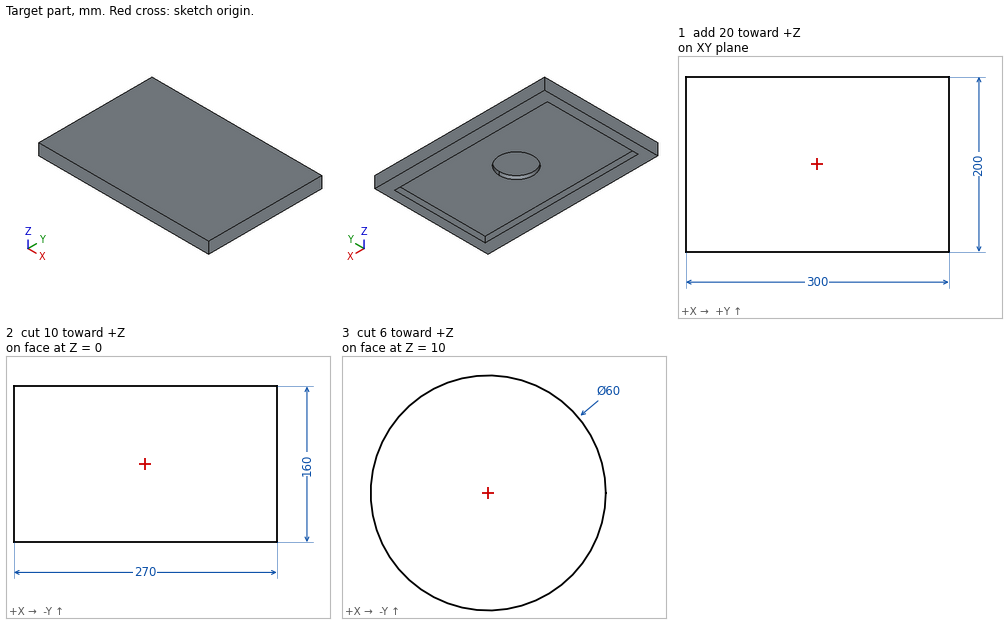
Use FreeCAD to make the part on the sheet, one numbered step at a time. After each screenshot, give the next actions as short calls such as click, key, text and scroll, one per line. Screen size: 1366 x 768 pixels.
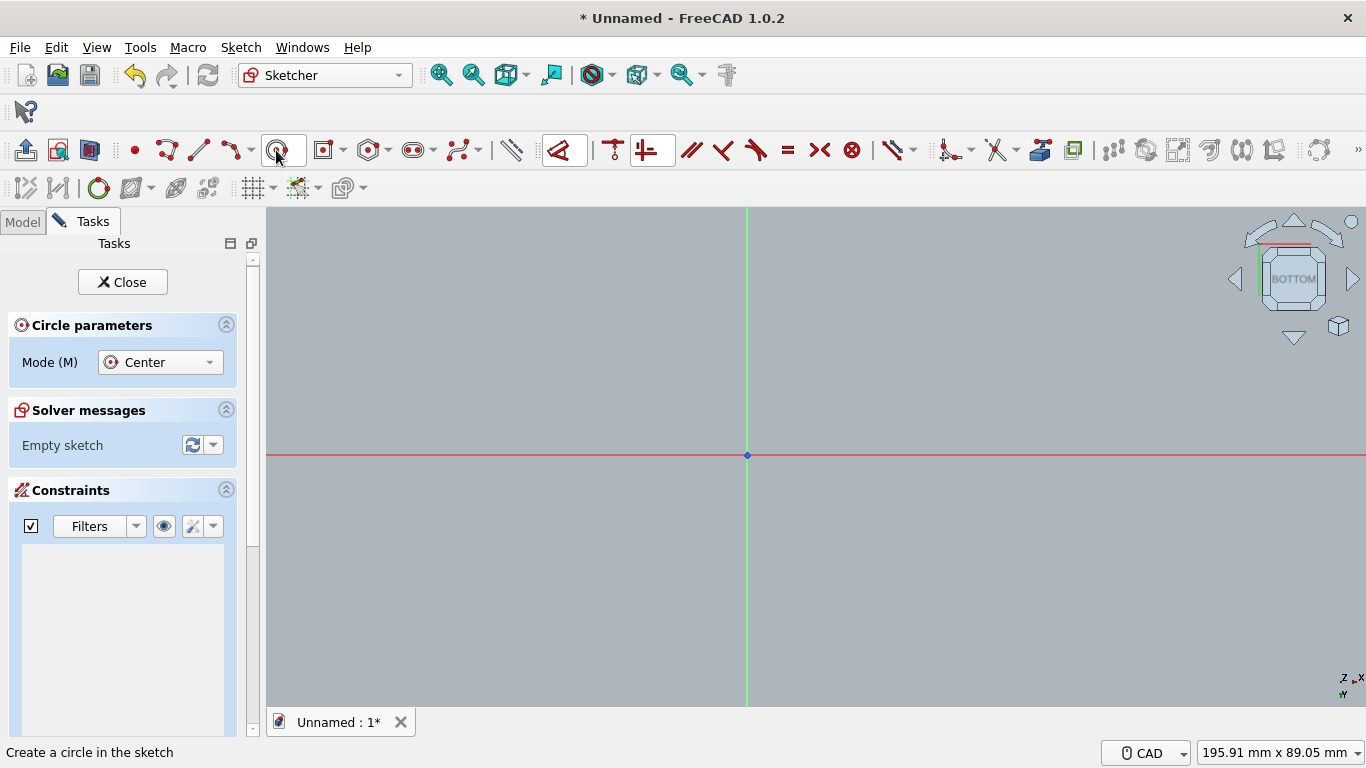
click(747, 455)
click(866, 336)
key(Escape)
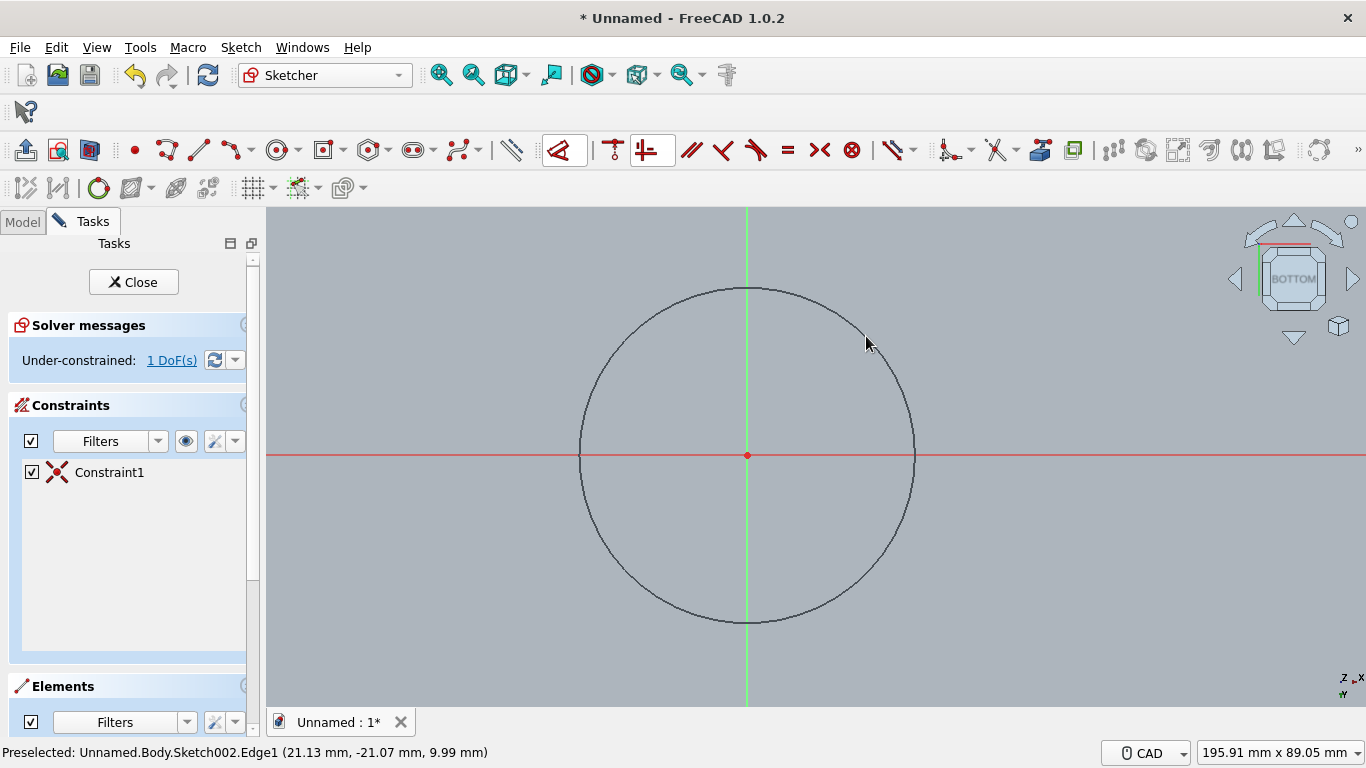
click(865, 336)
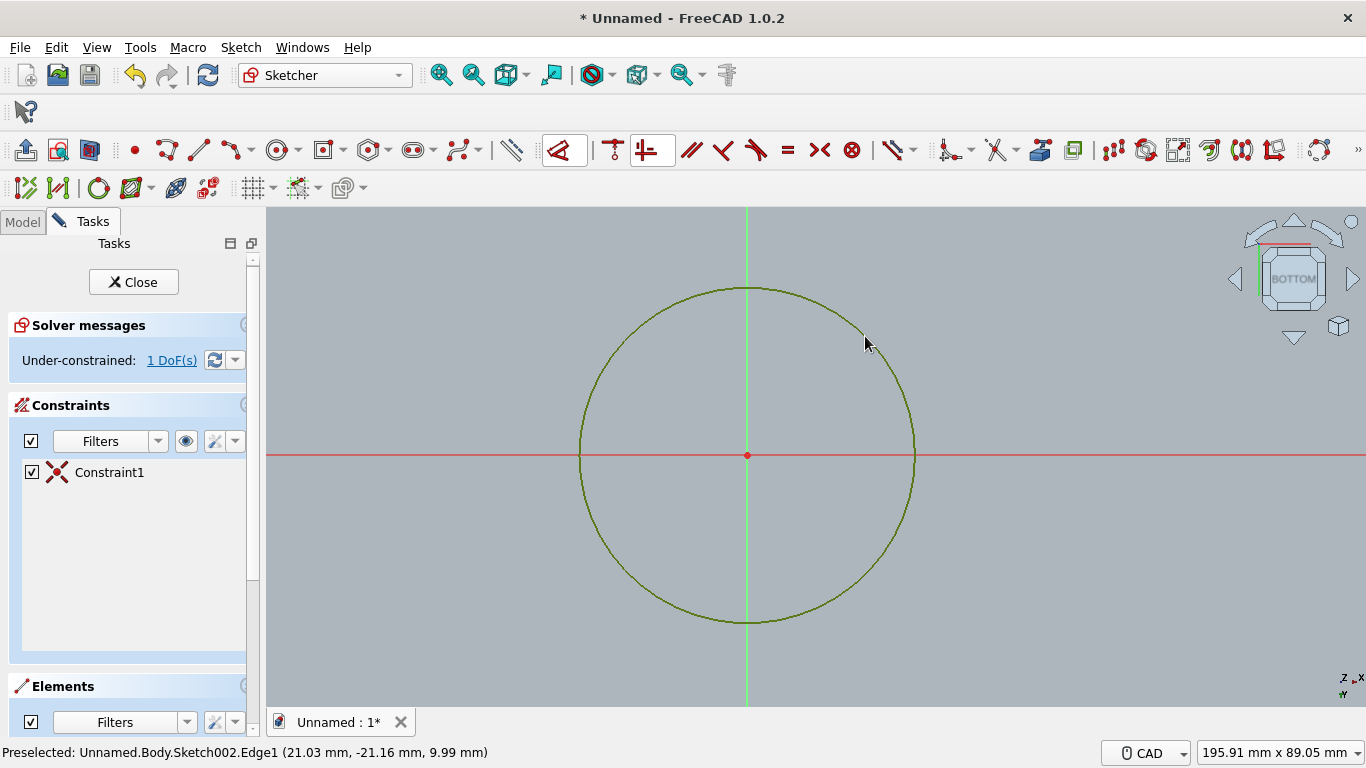
key(k)
key(o)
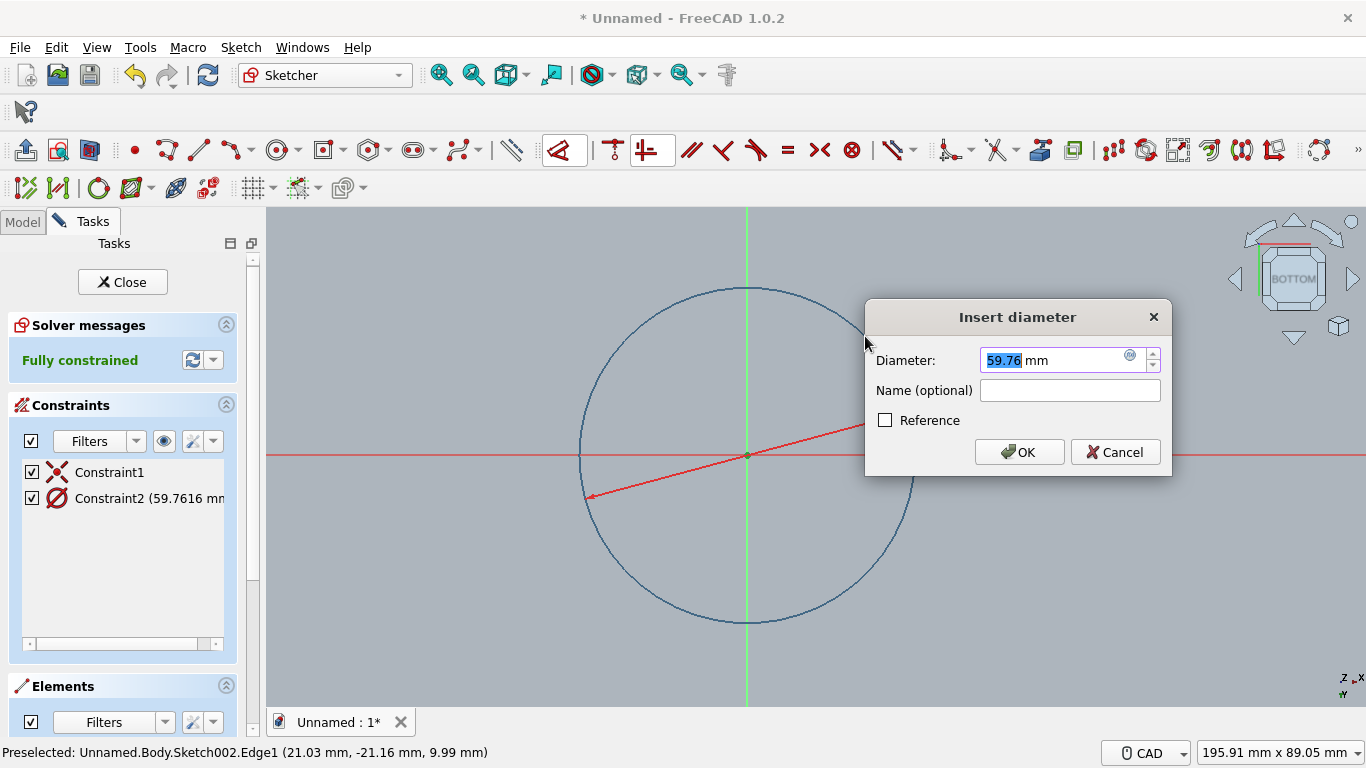
text(60)
key(Return)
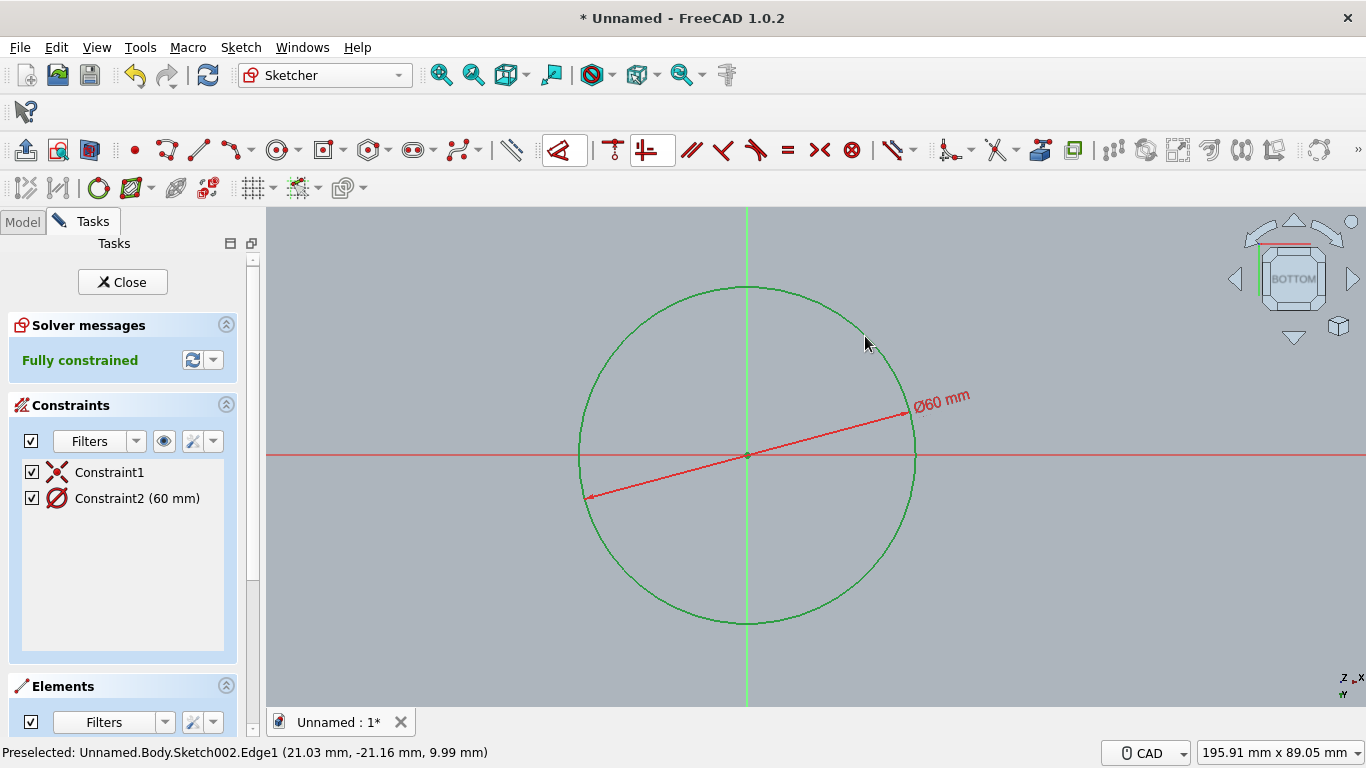
click(123, 282)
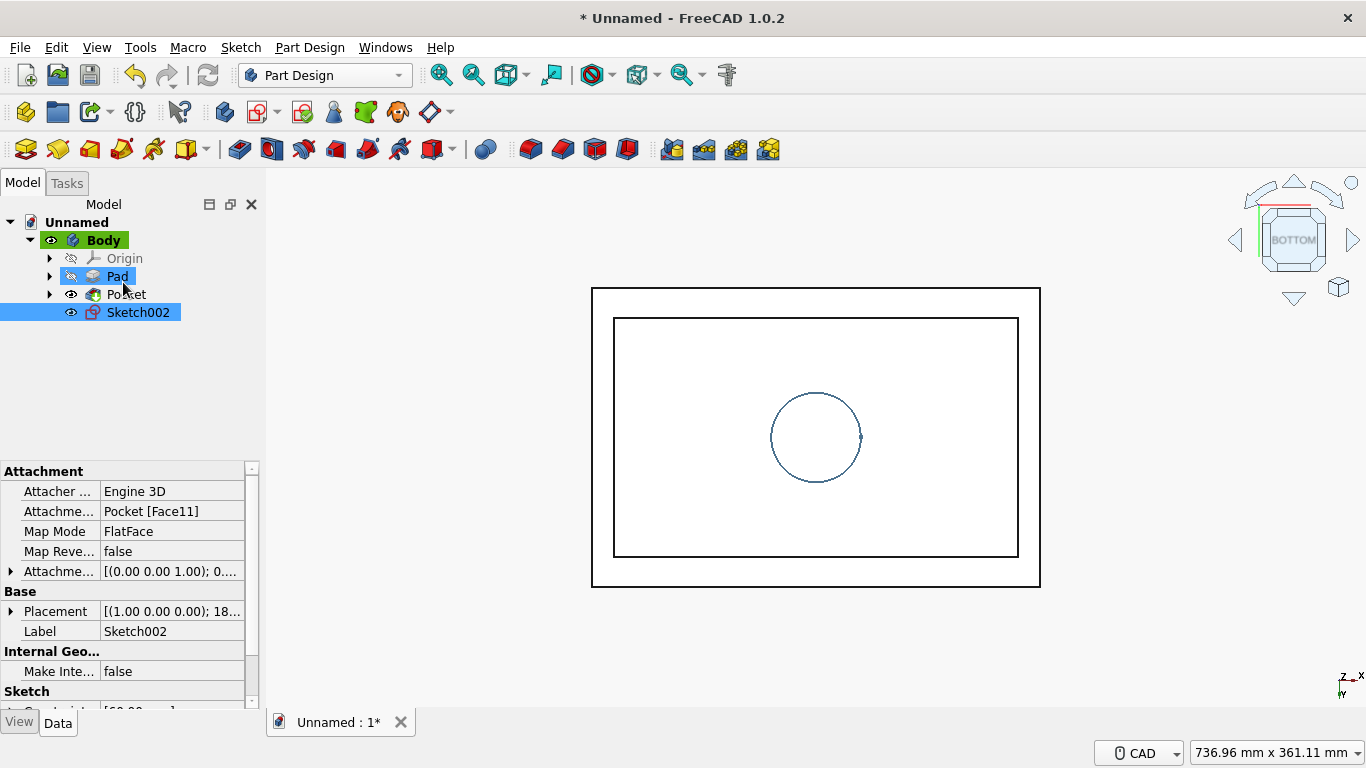
click(240, 150)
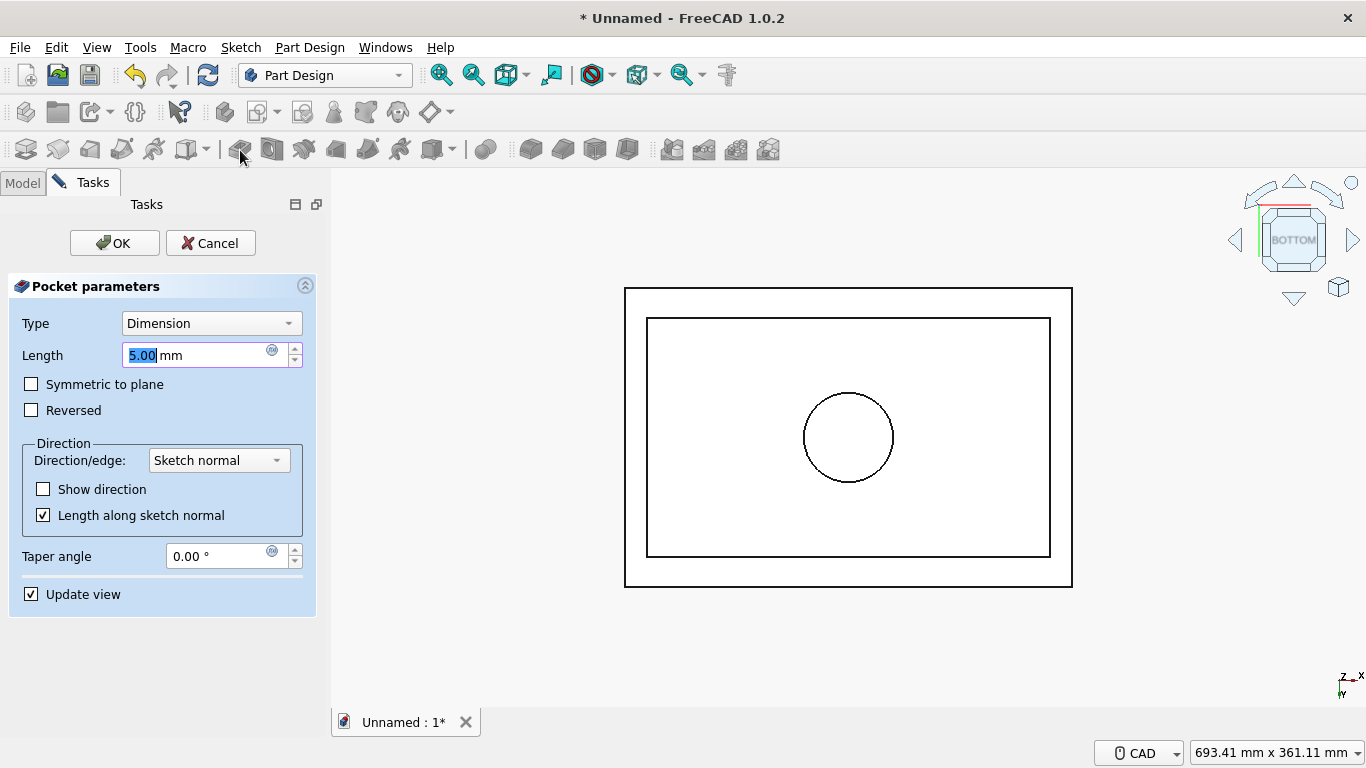
text(6)
key(Tab)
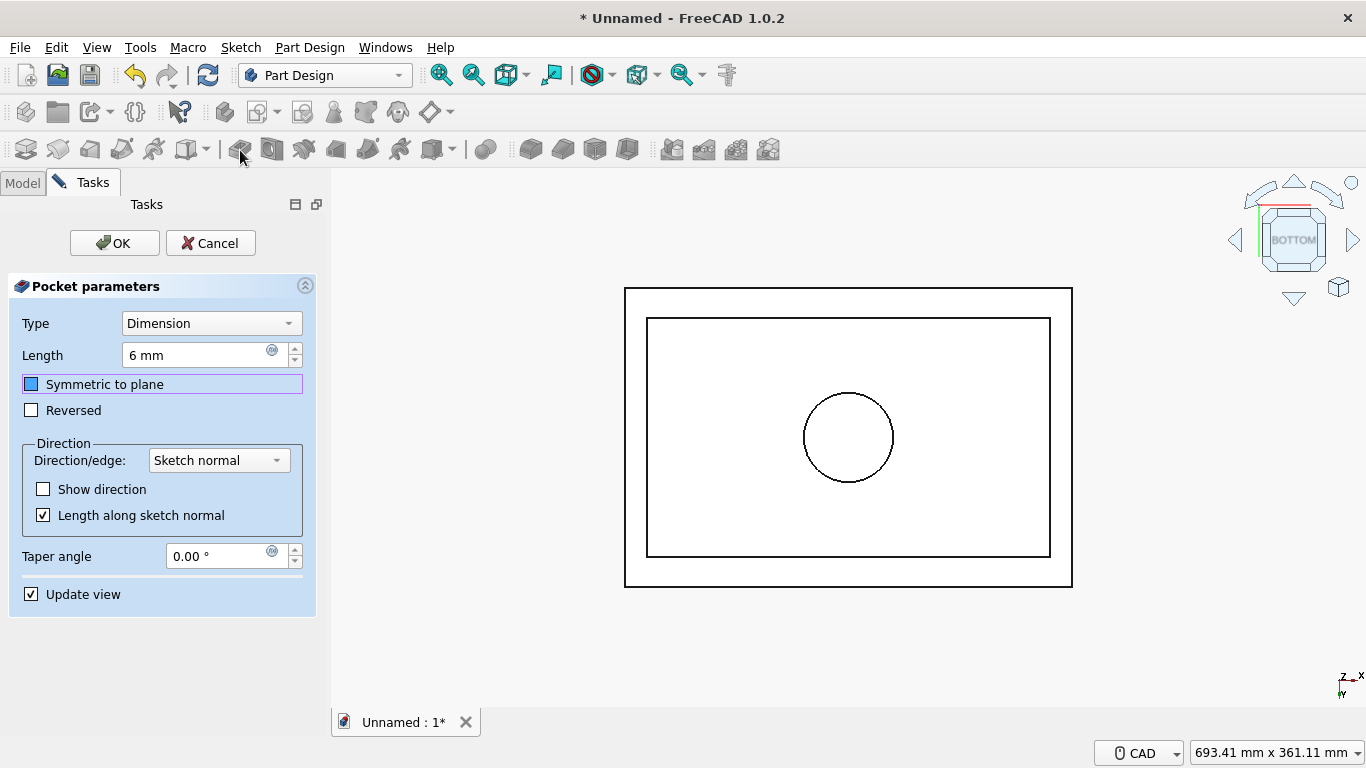
click(115, 243)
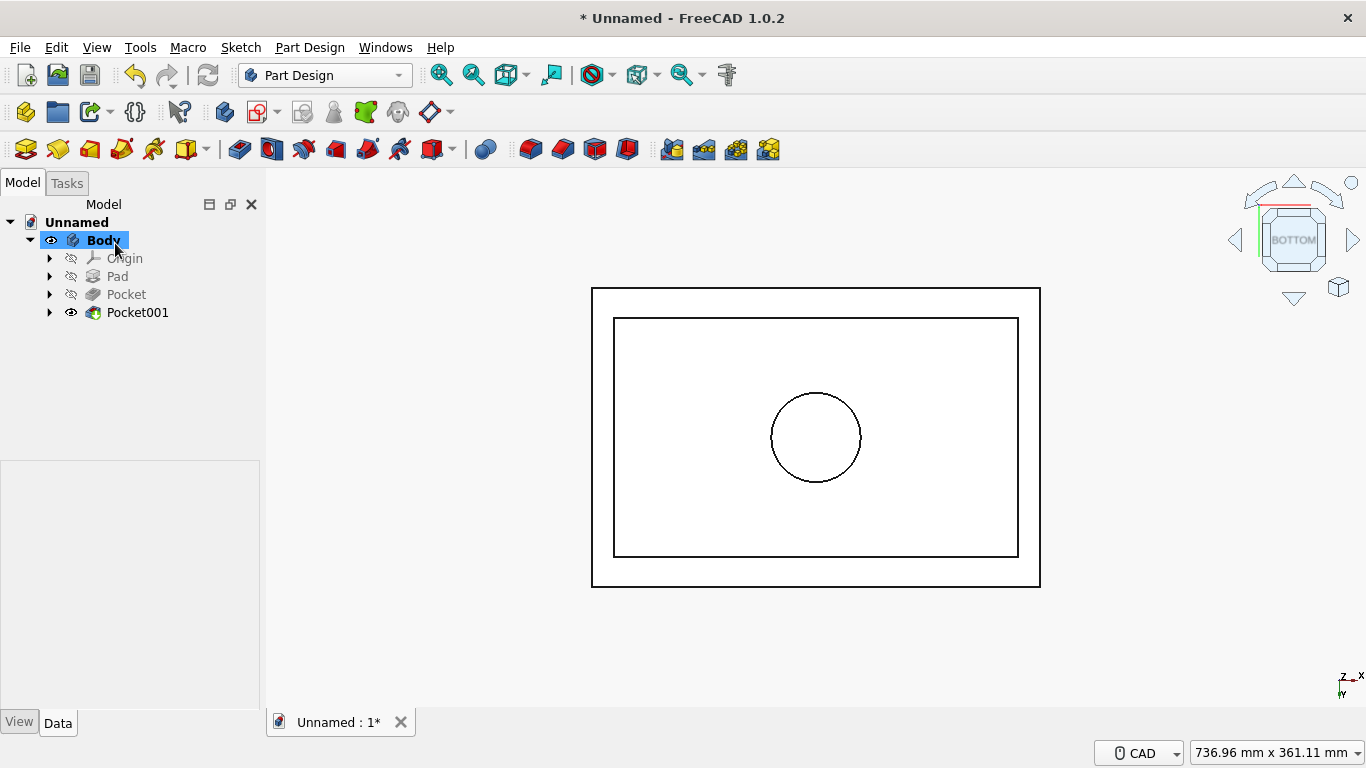
key(0)